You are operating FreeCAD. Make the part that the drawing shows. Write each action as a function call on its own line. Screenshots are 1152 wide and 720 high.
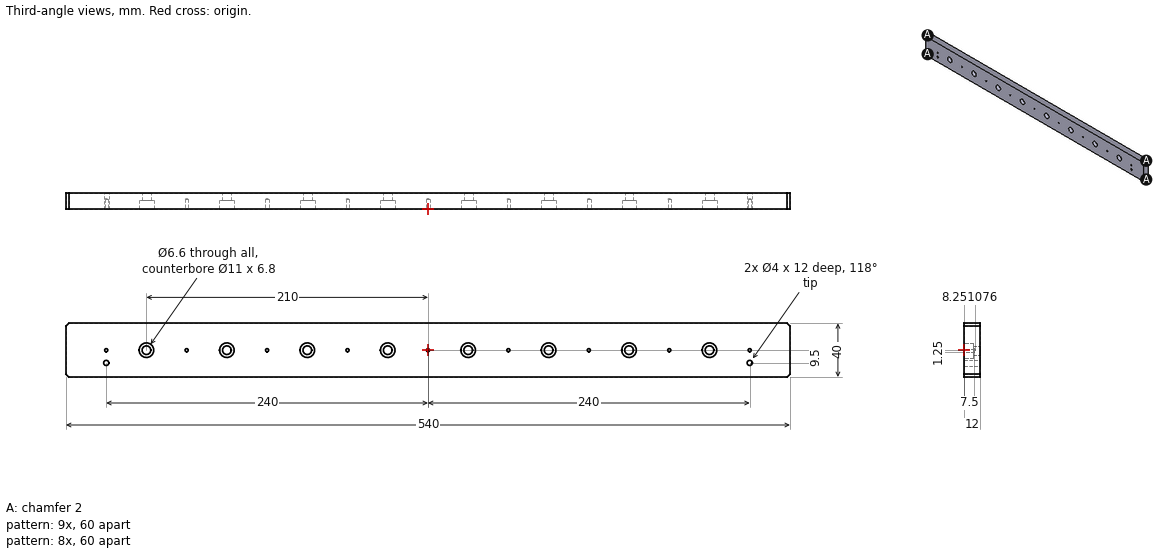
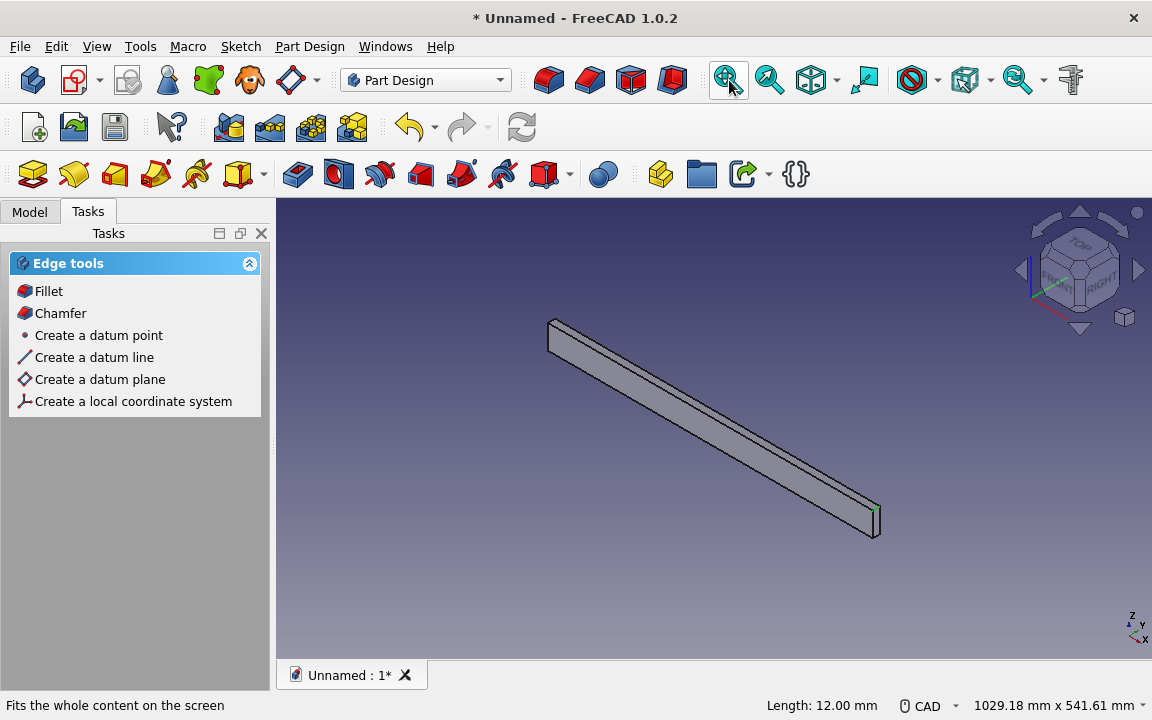
key(2)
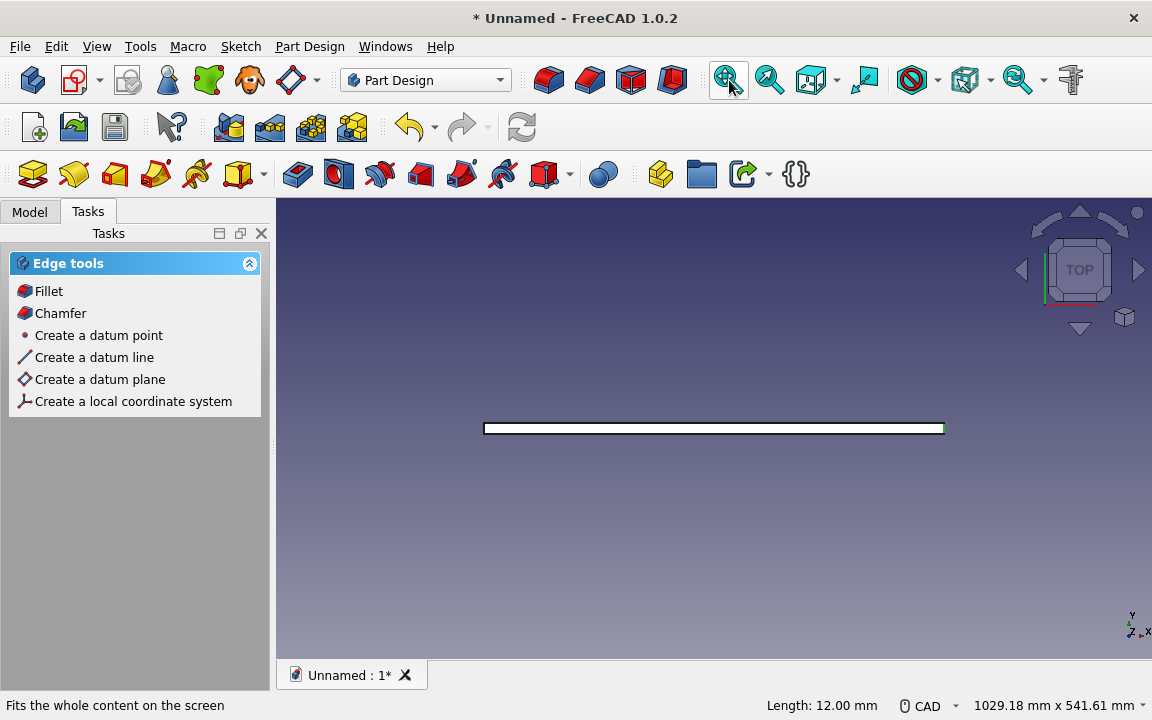
click(484, 429, ctrl)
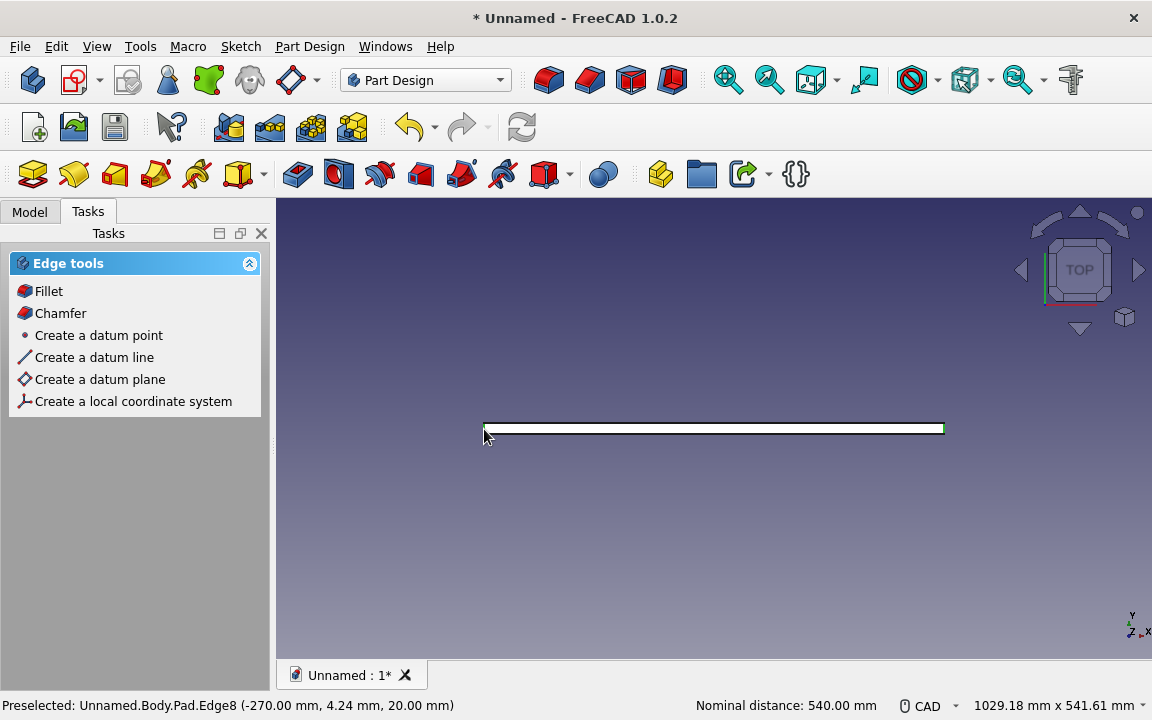
scroll(484, 427, up, 7)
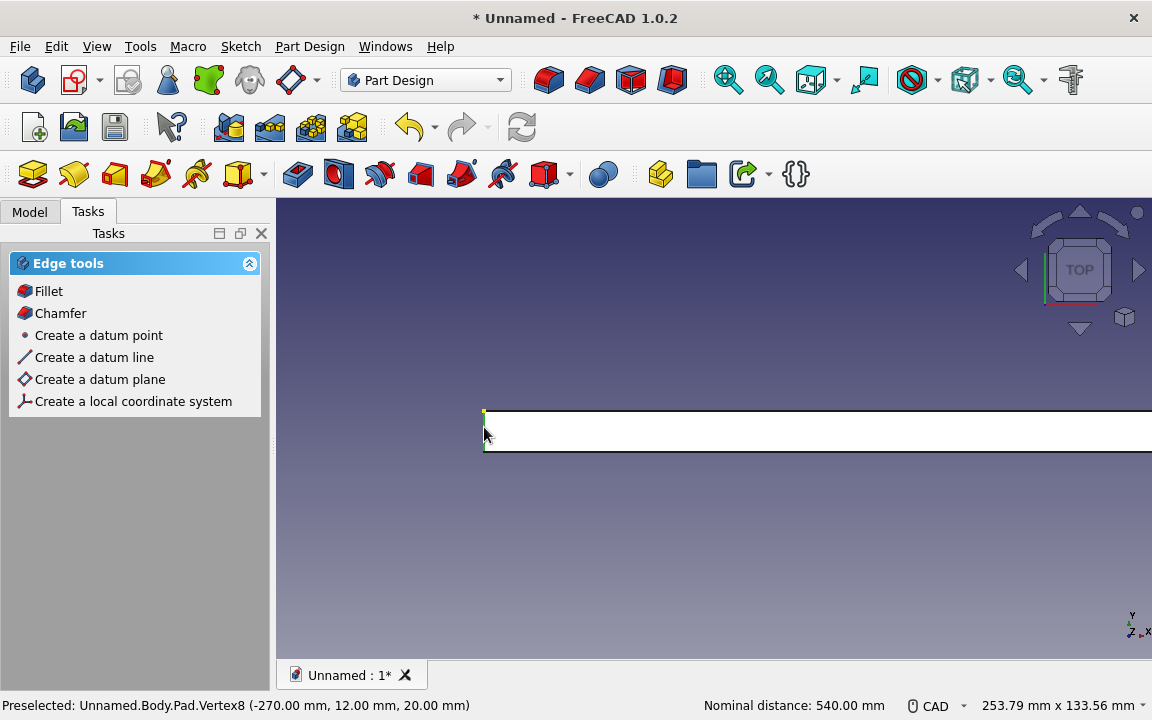
click(729, 80)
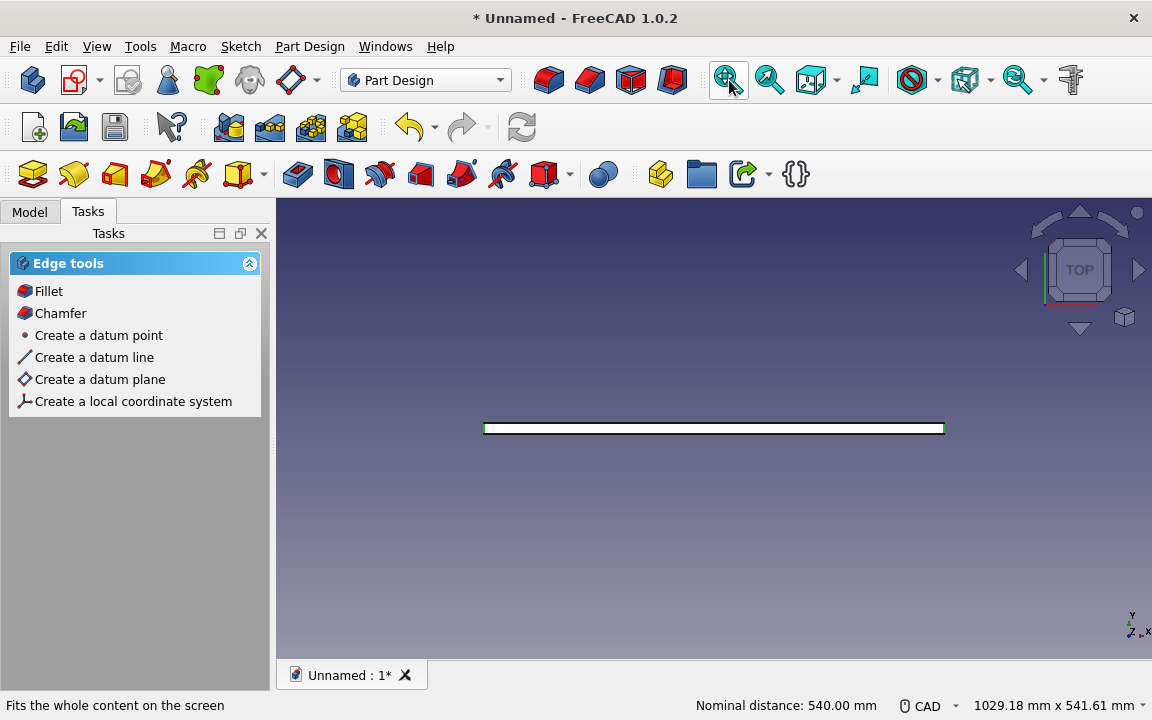
key(1)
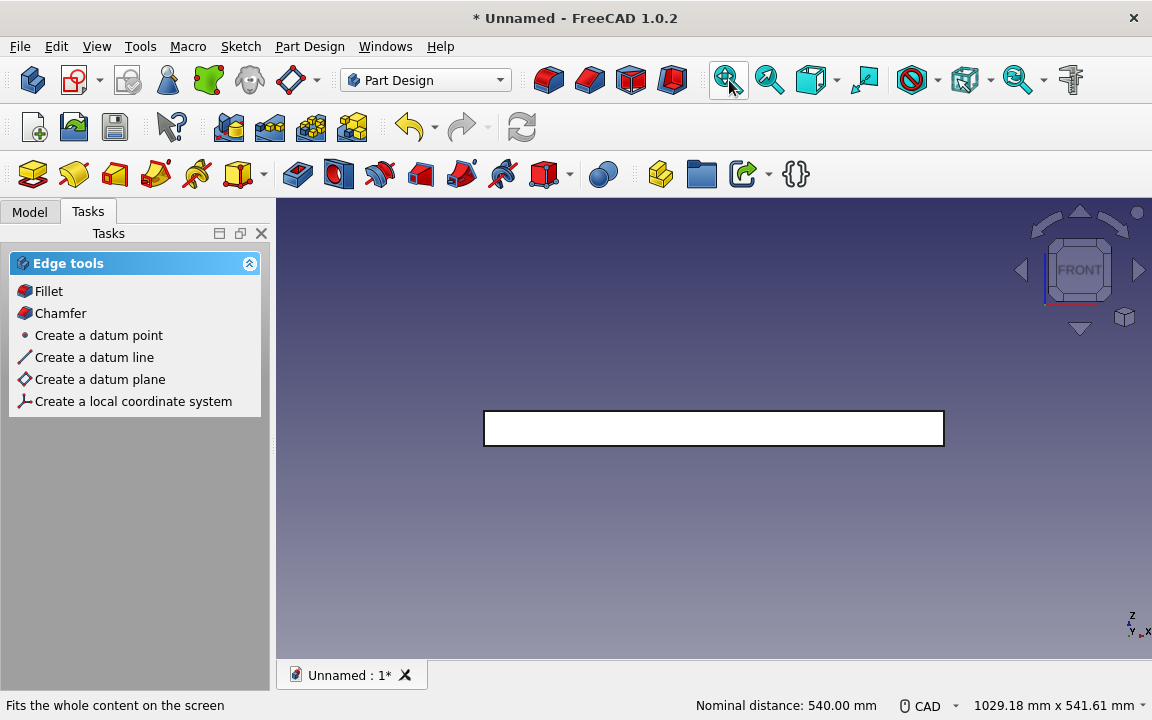
scroll(484, 445, up, 7)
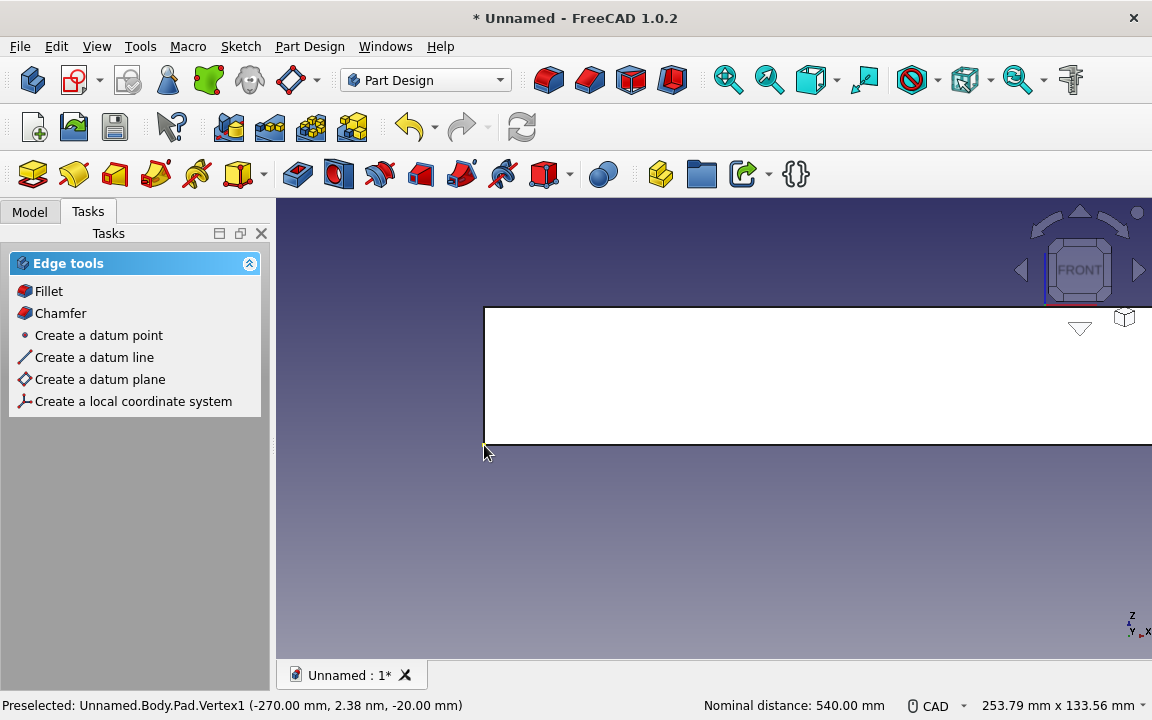
click(729, 80)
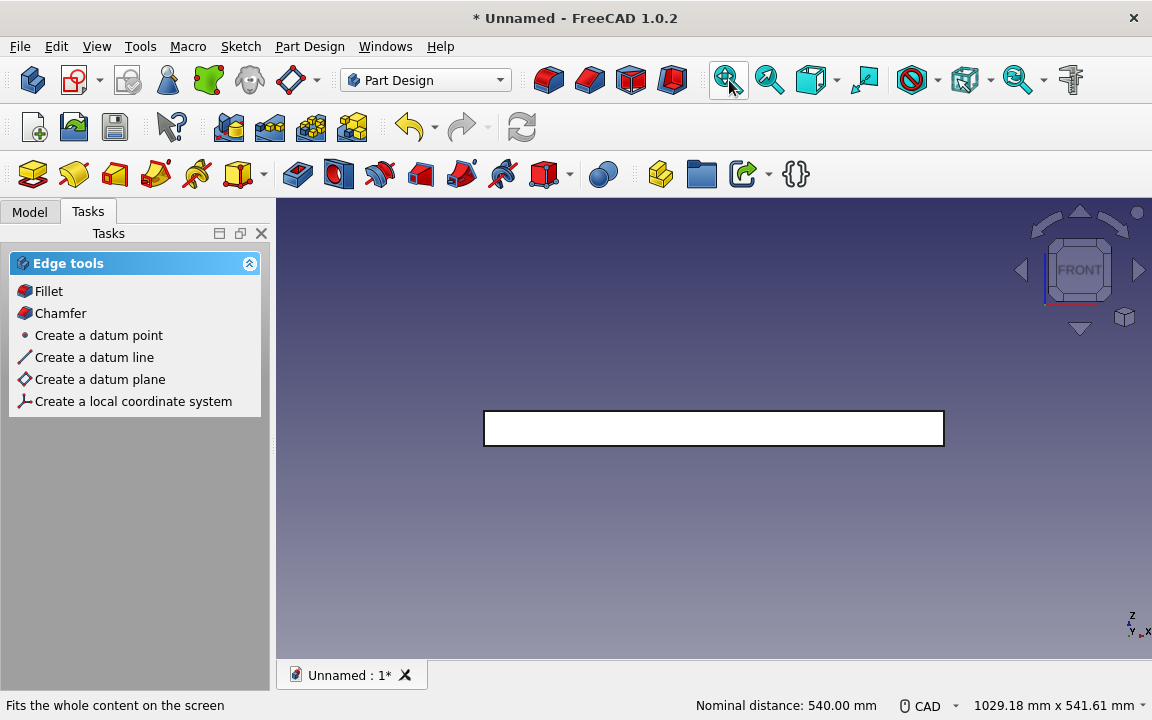
key(3)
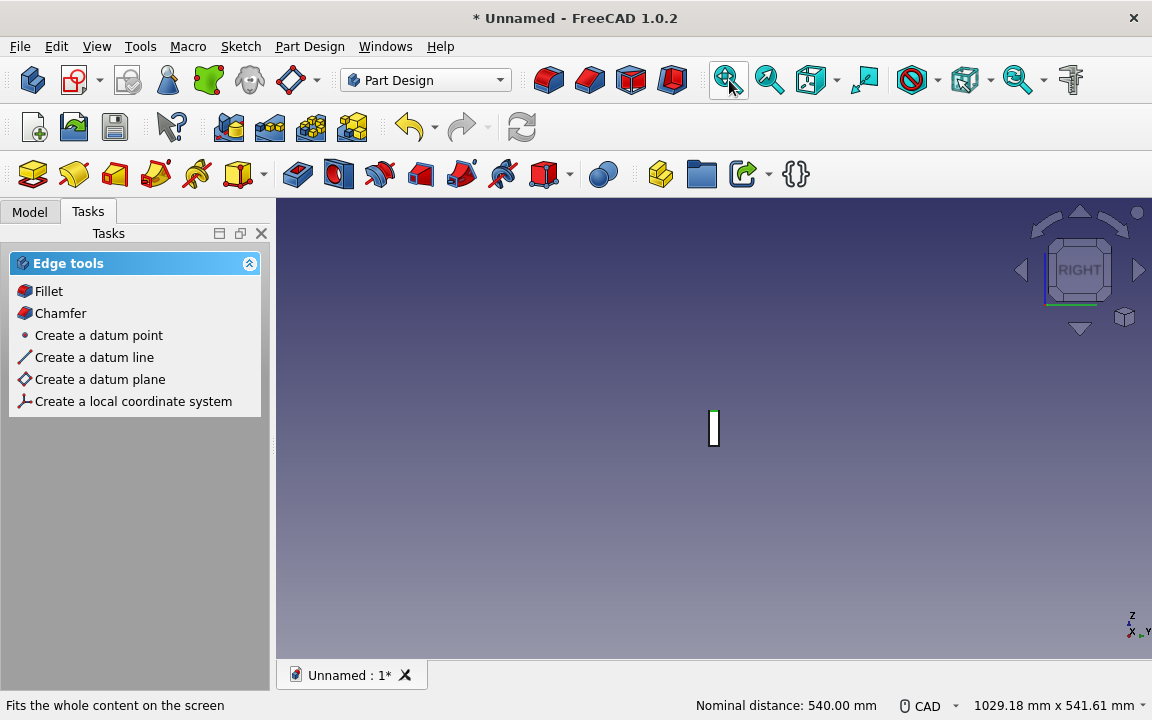
click(729, 80)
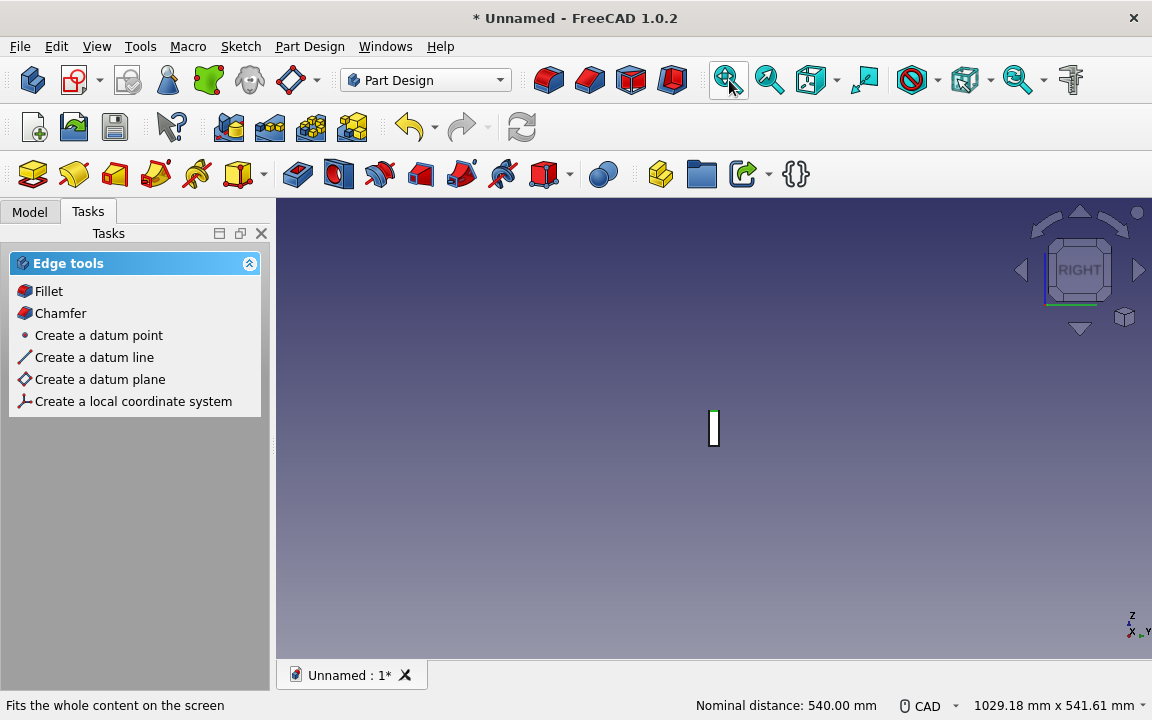
scroll(714, 445, up, 7)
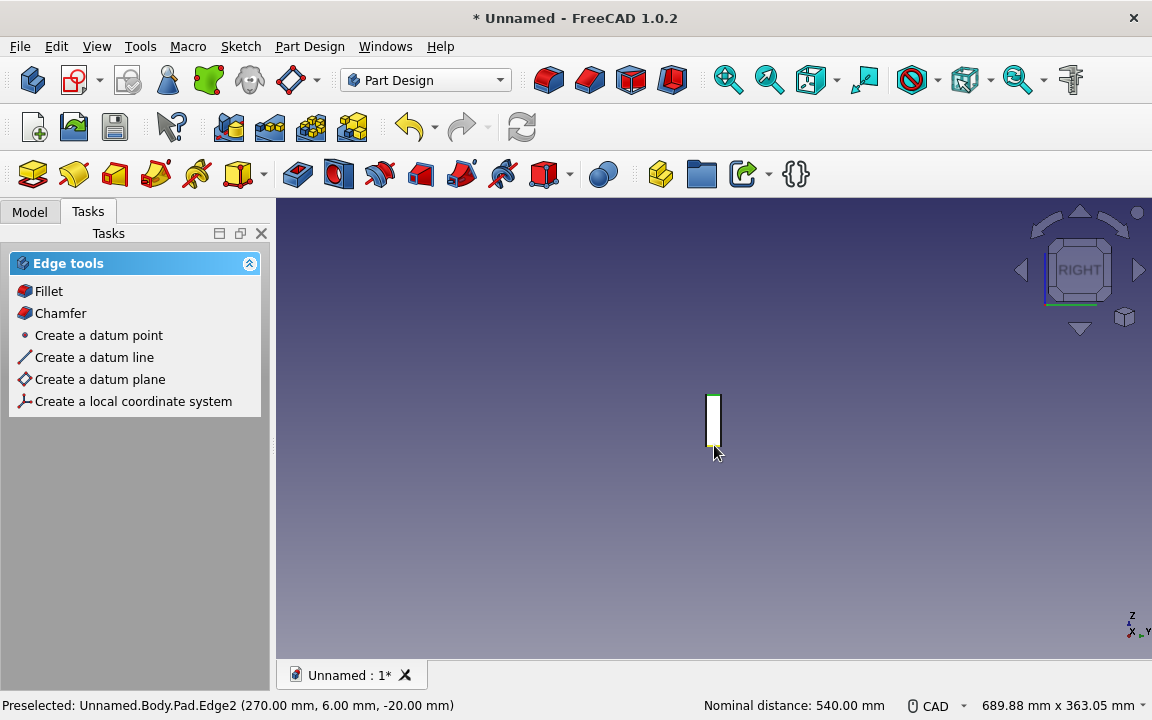
click(712, 444, ctrl)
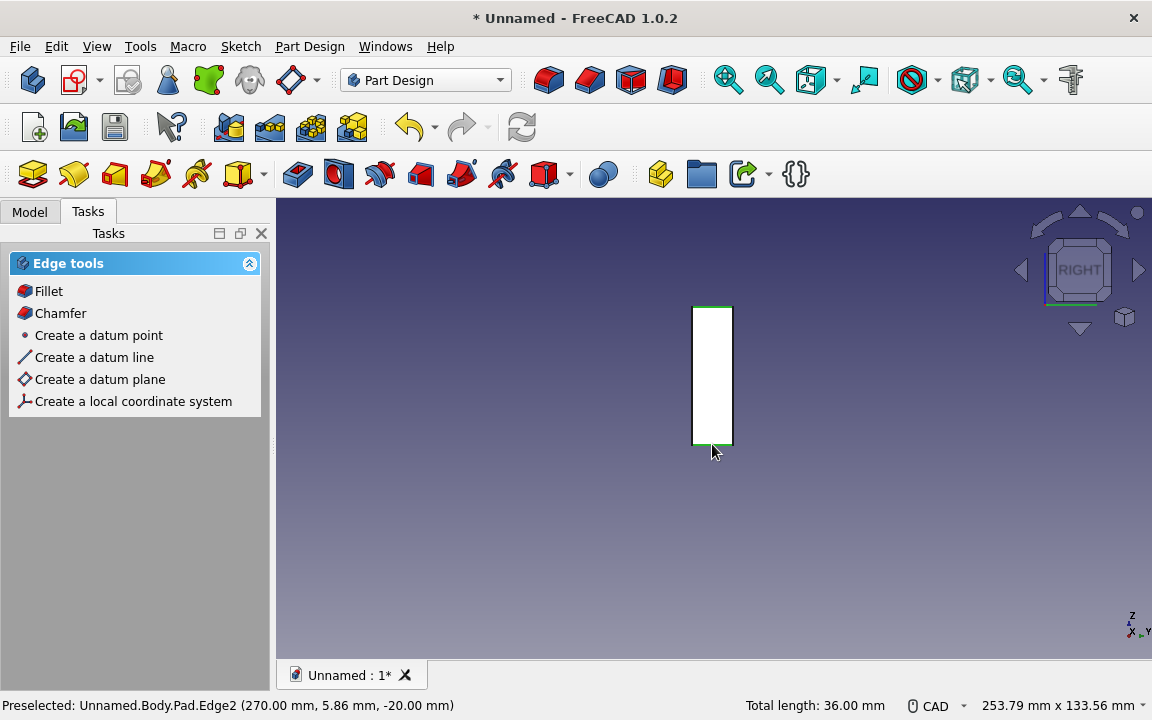
key(v)
key(f)